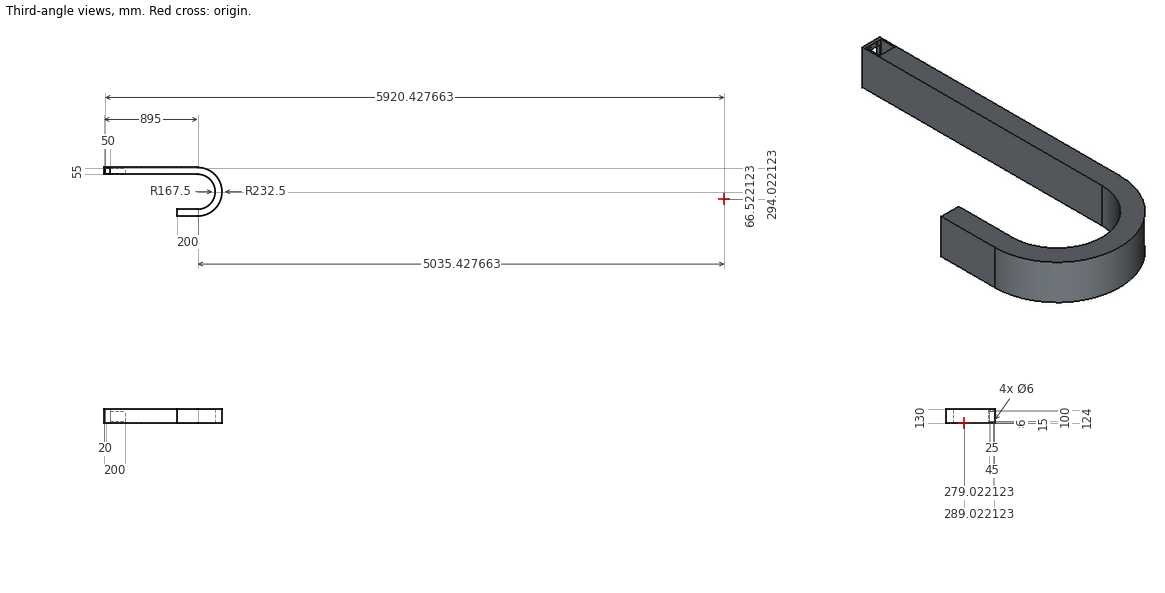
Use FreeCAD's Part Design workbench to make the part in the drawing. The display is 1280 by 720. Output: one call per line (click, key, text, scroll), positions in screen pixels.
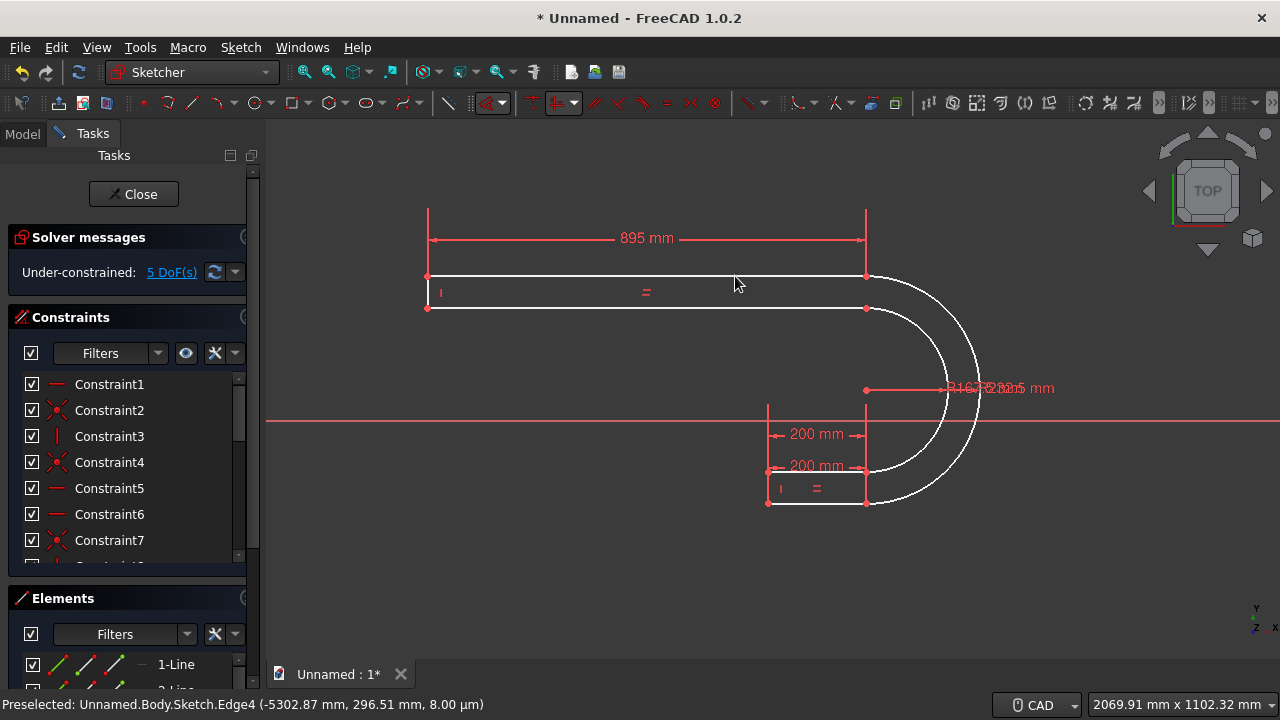
click(559, 308)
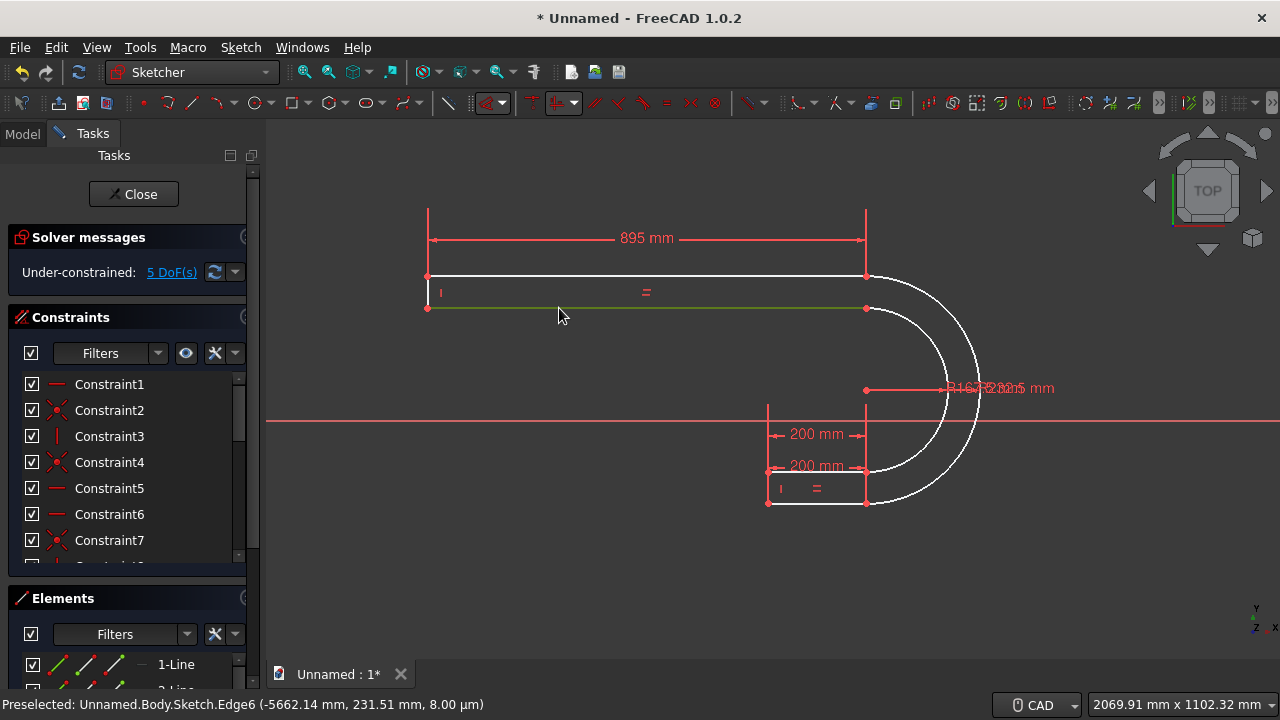
key(l)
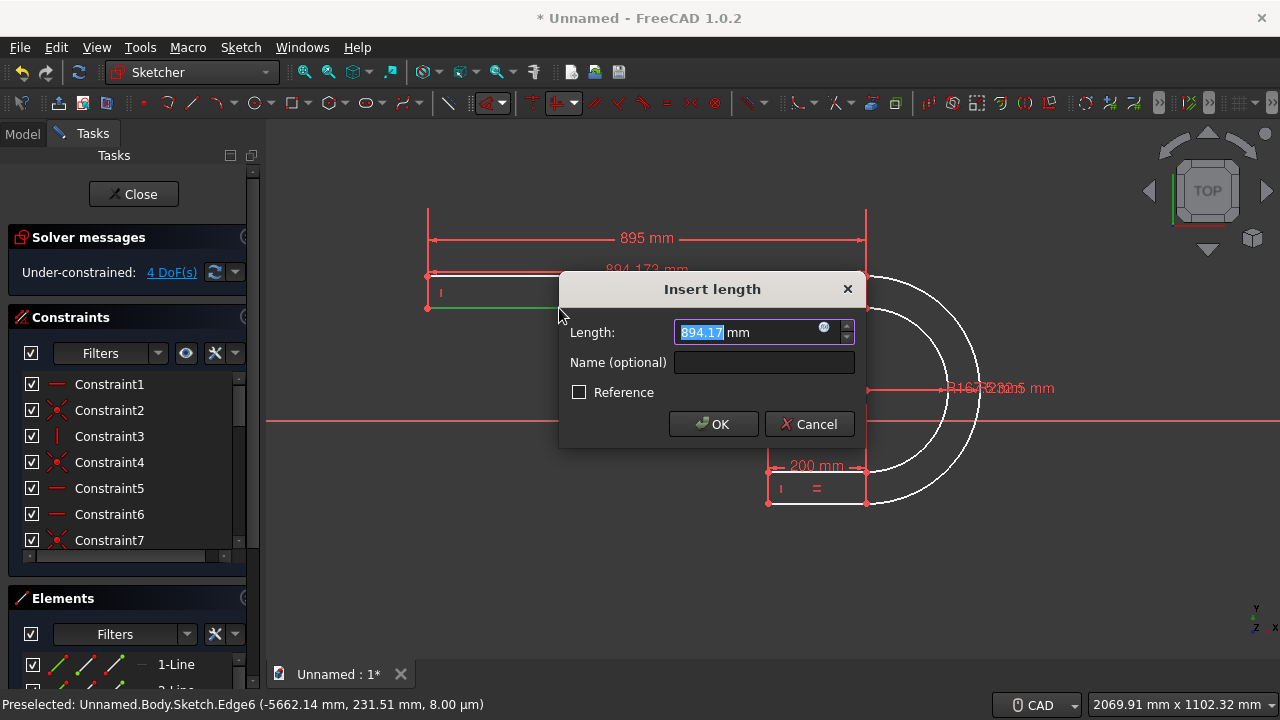
text(895)
key(Return)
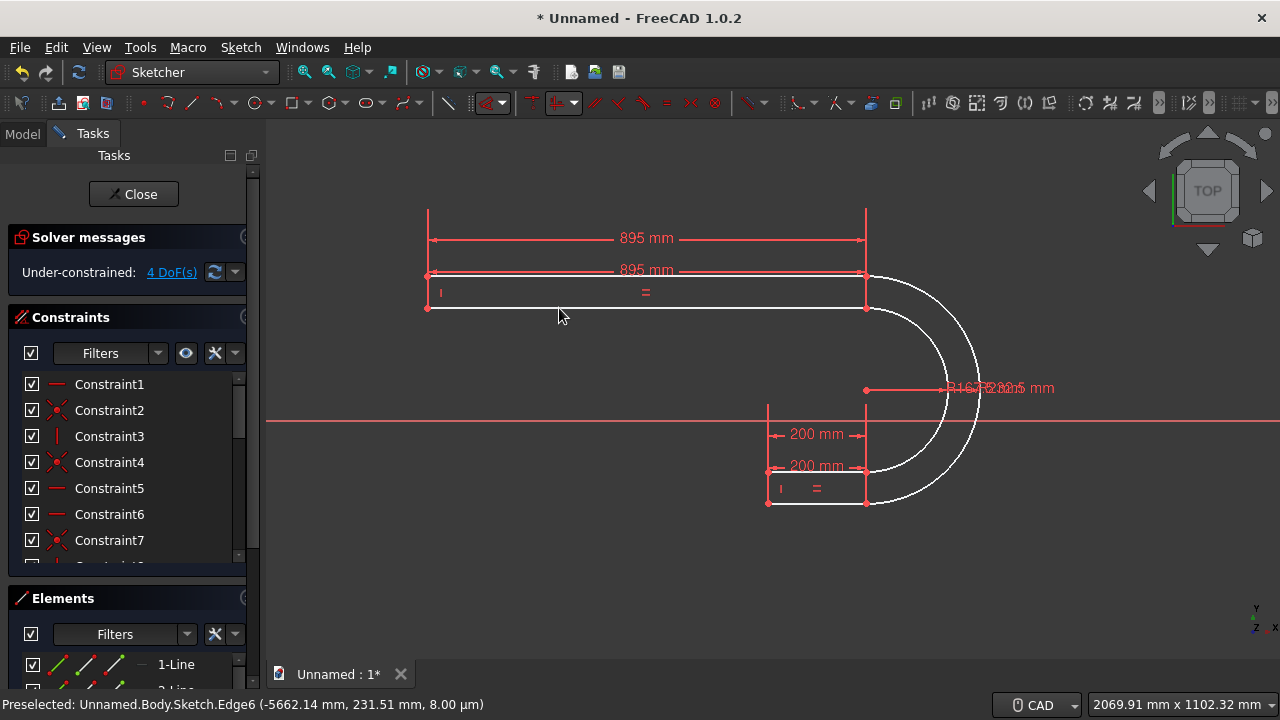
click(866, 390)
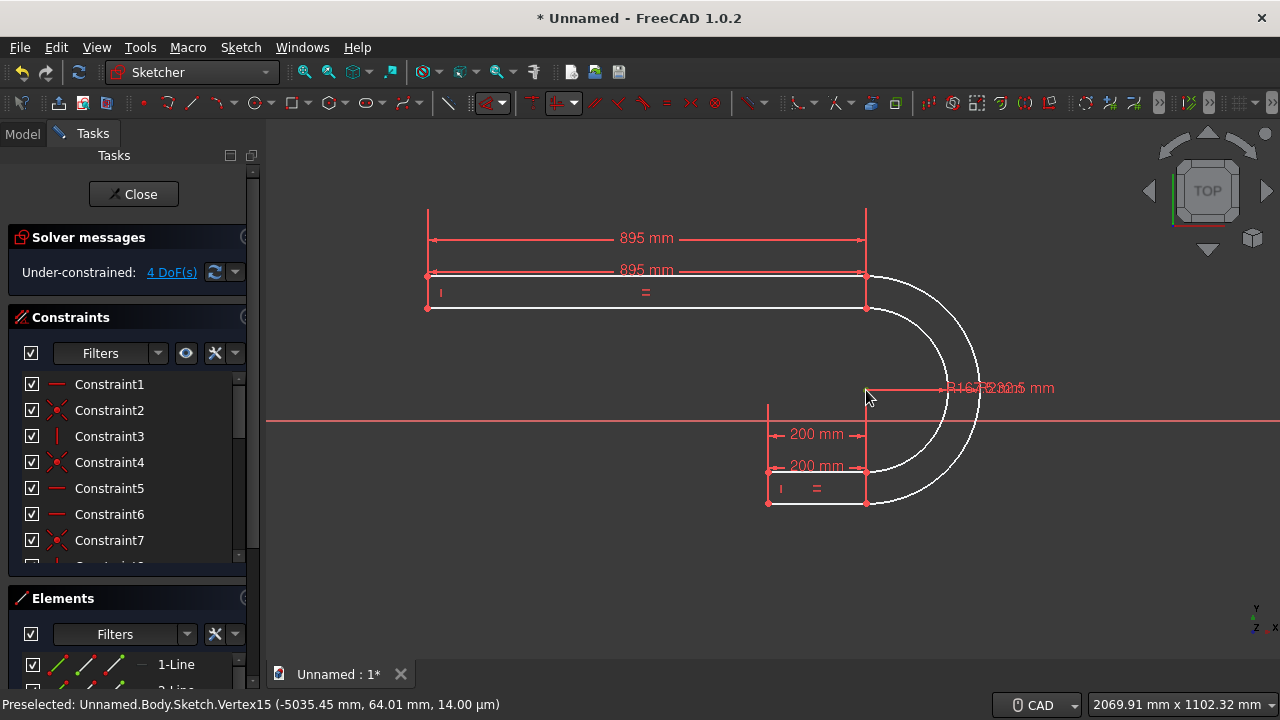
key(i)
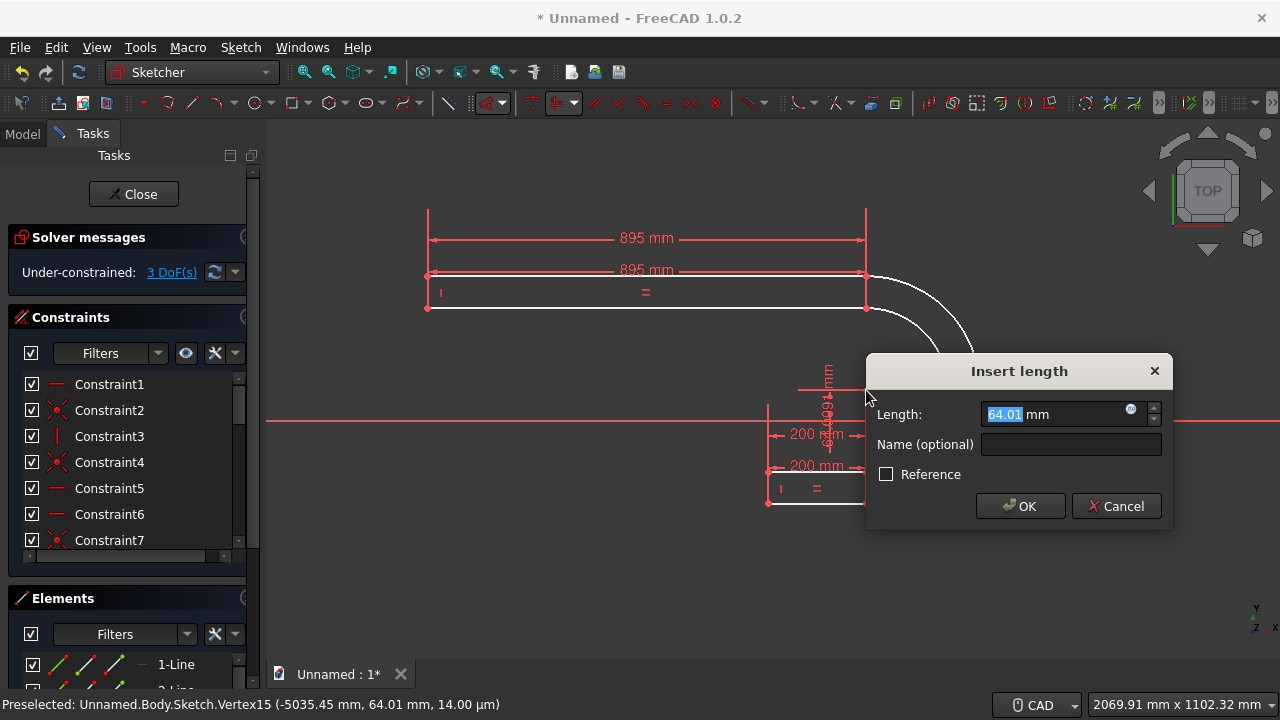
text(66.522123)
key(Return)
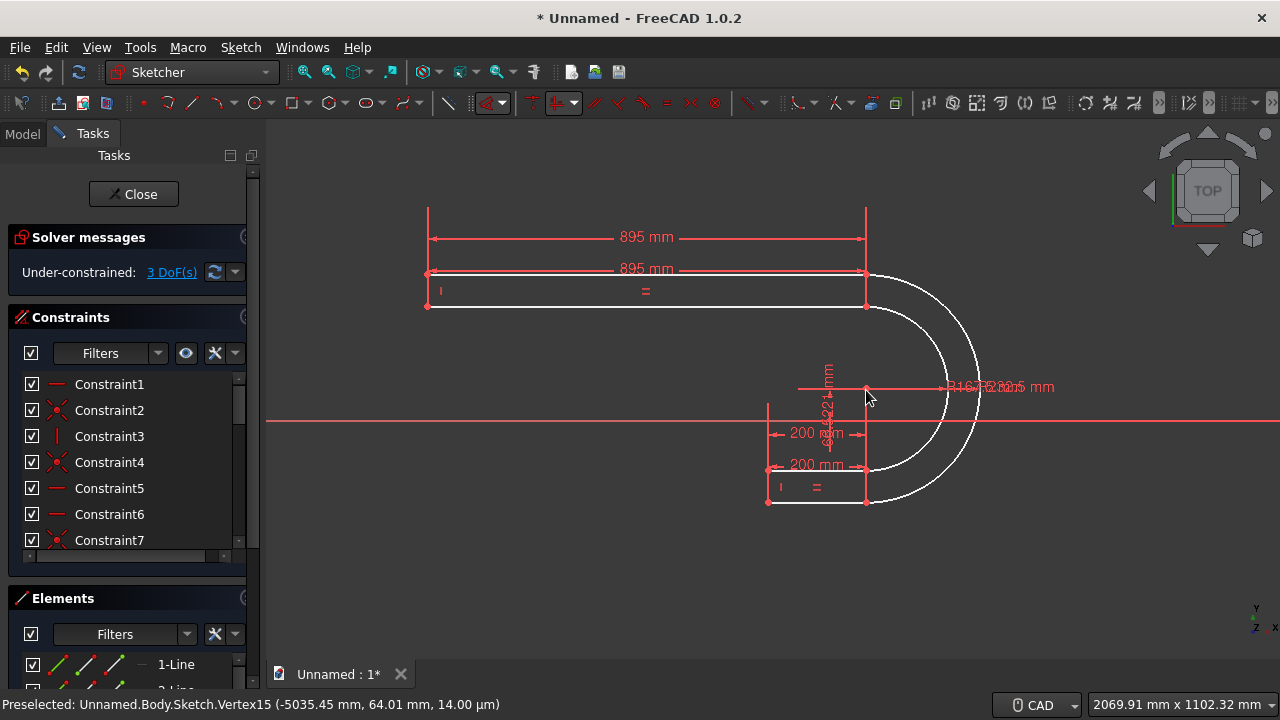
click(866, 471)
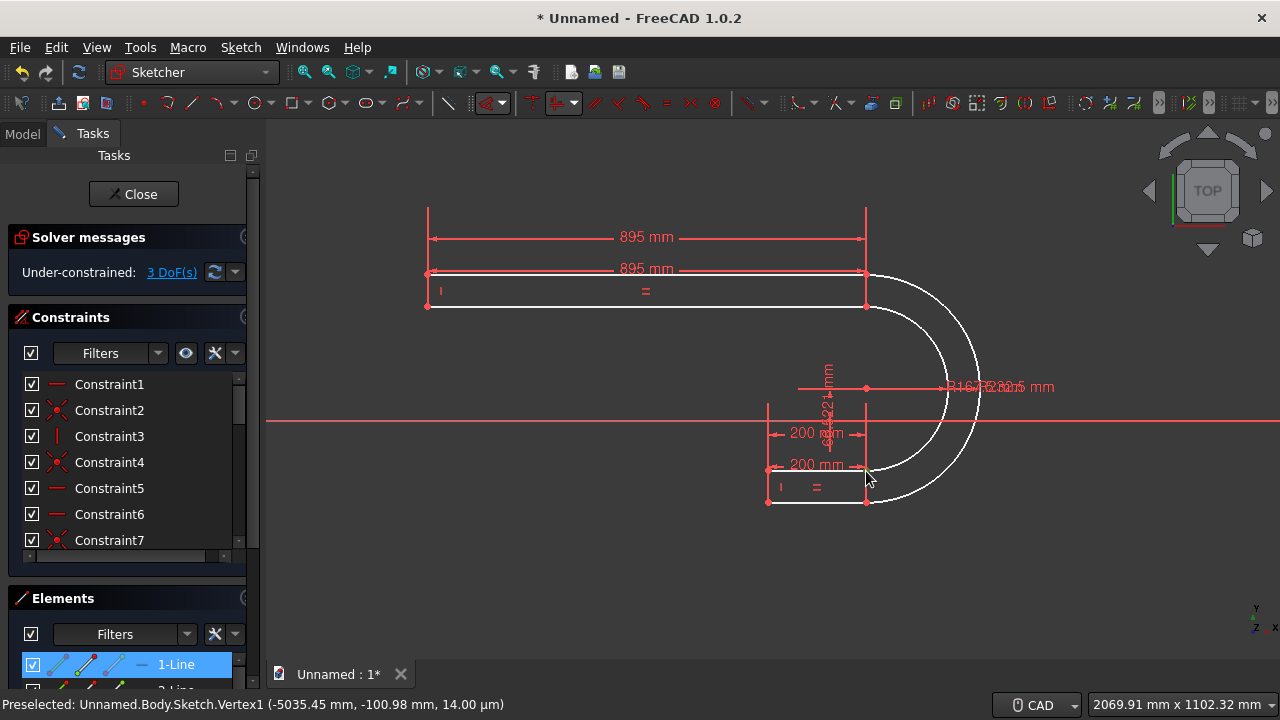
key(l)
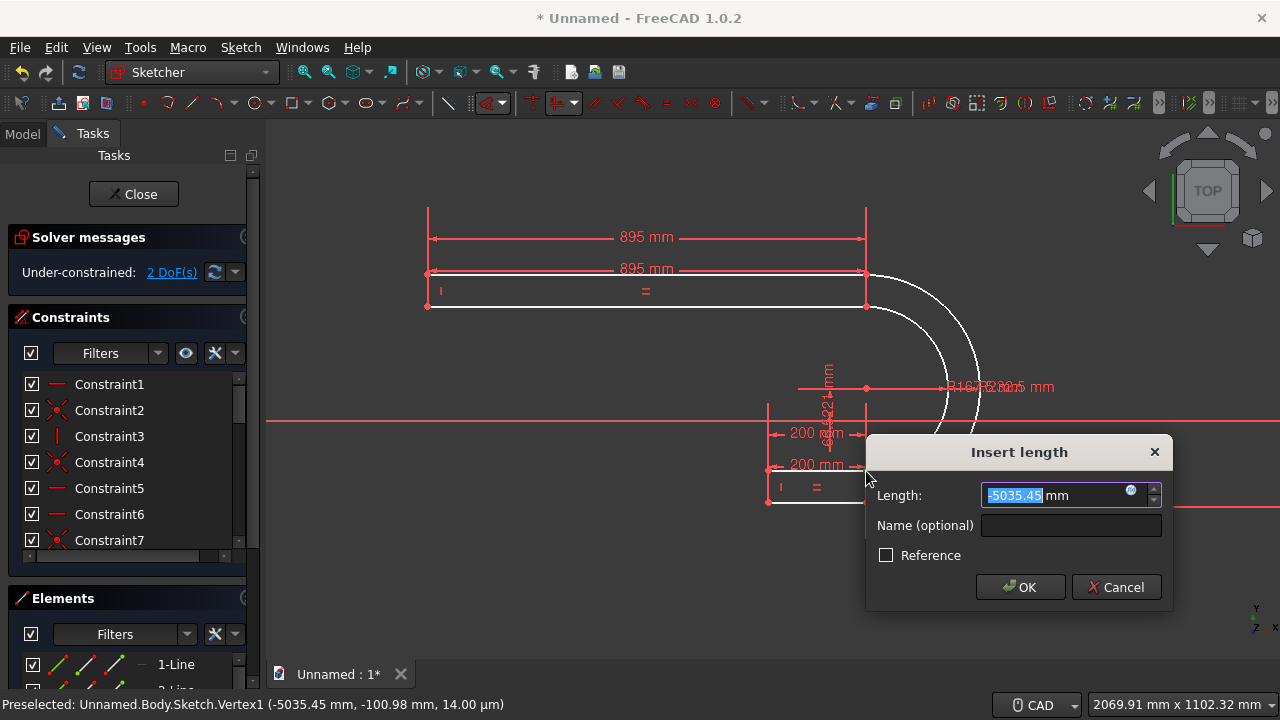
text(-5035.427663)
key(Return)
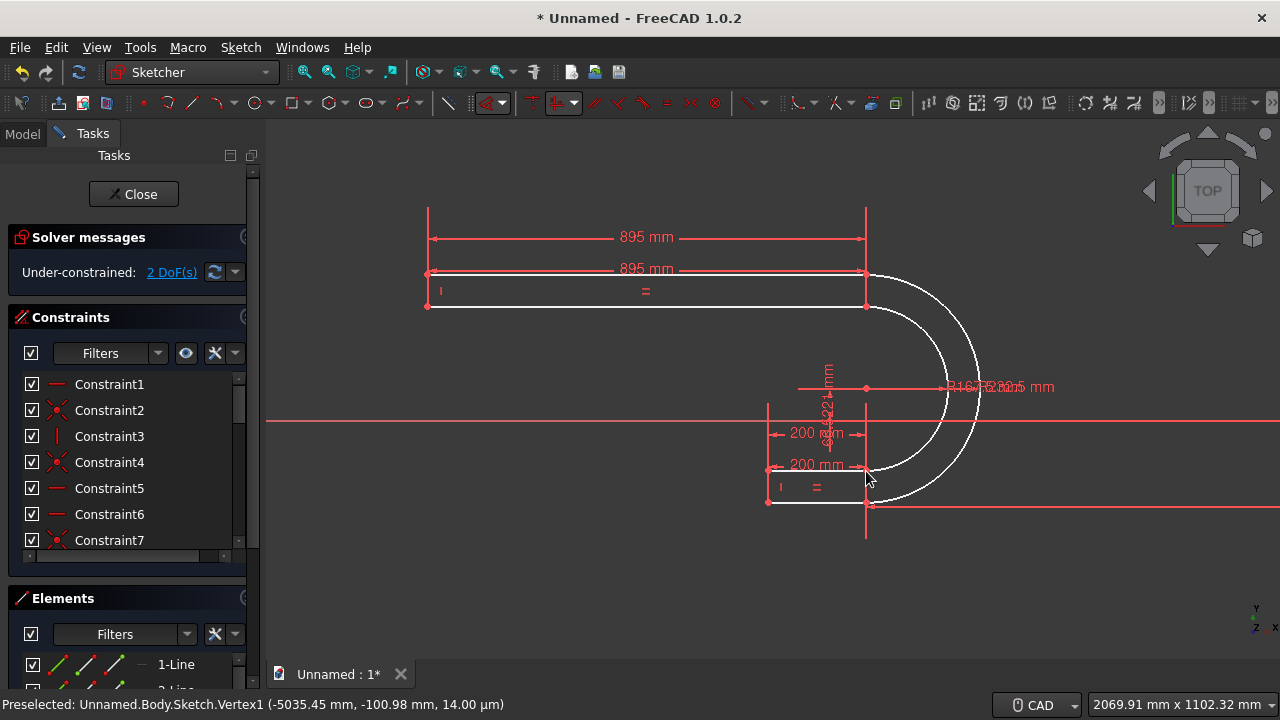
click(866, 275)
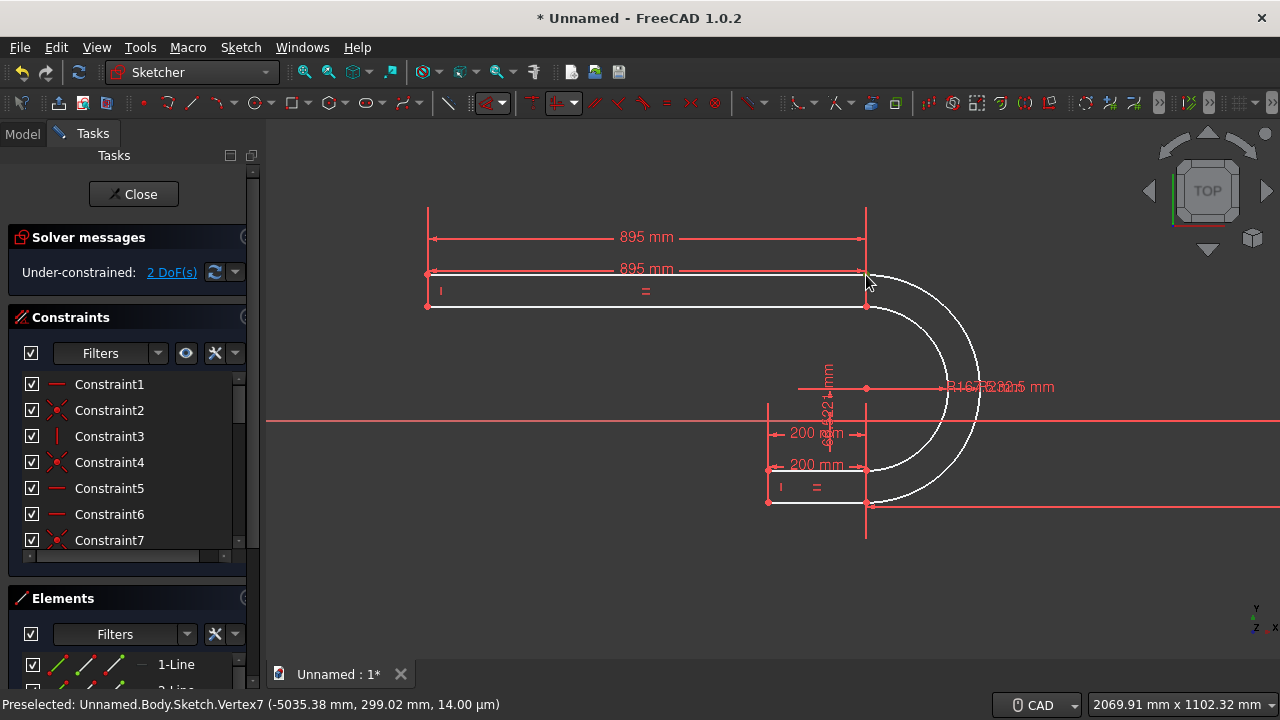
click(504, 104)